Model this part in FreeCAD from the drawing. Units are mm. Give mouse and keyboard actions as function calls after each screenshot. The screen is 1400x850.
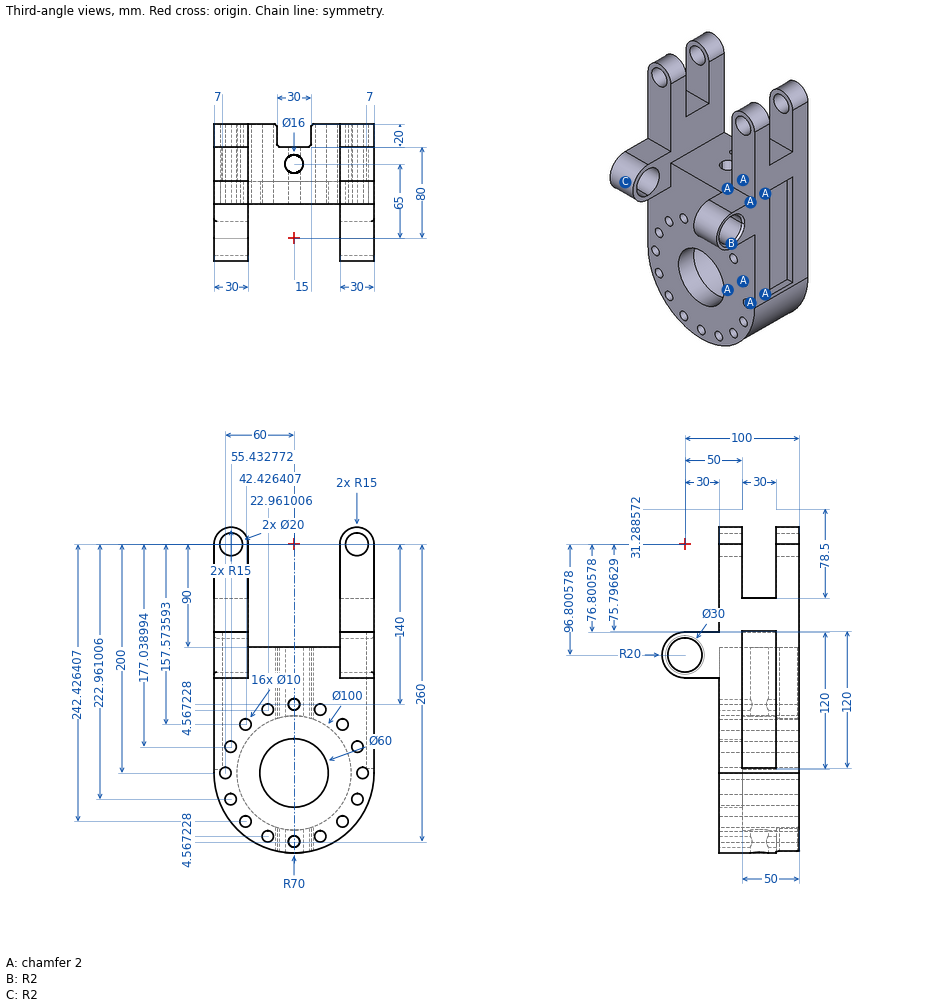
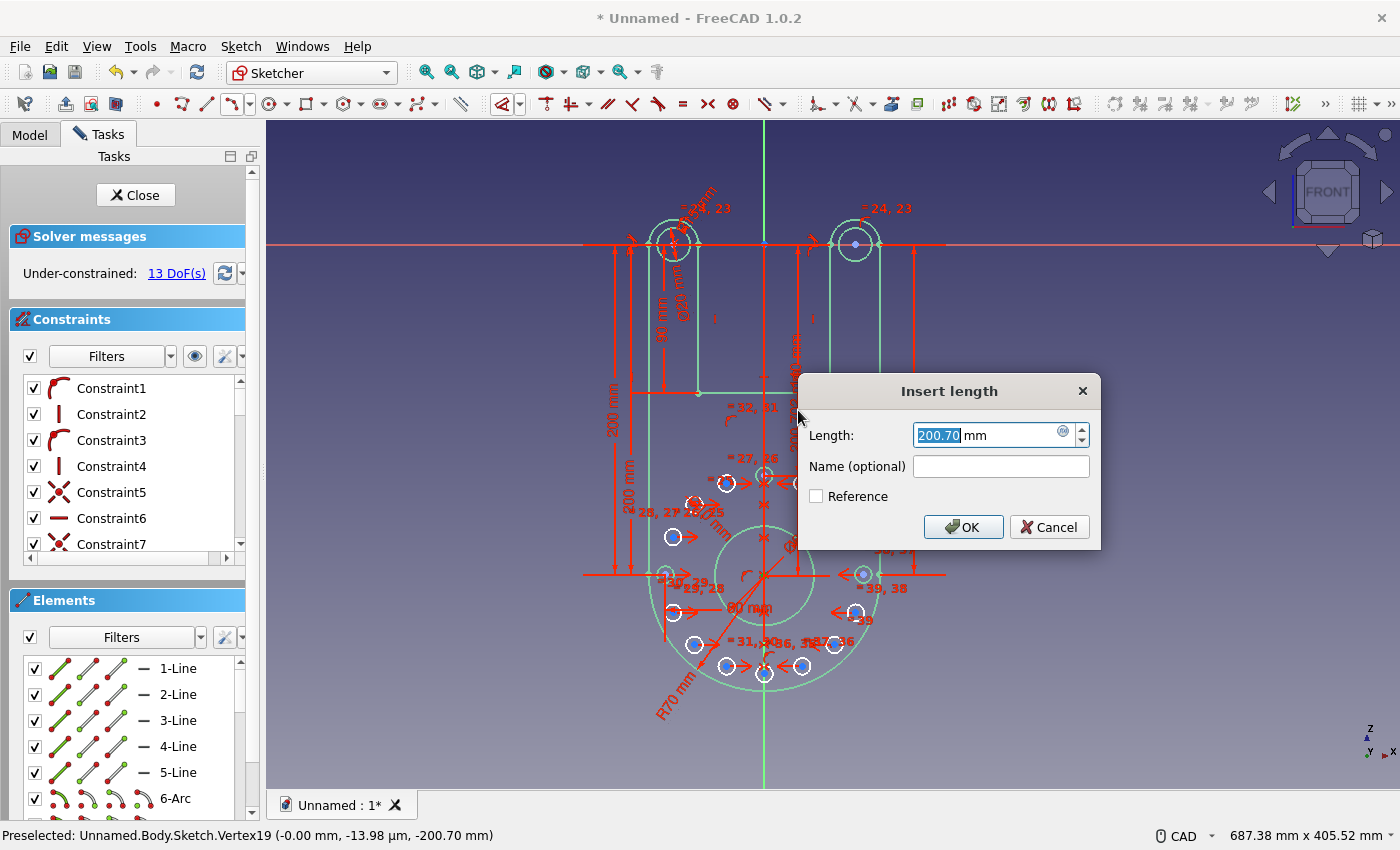
text(200)
key(Return)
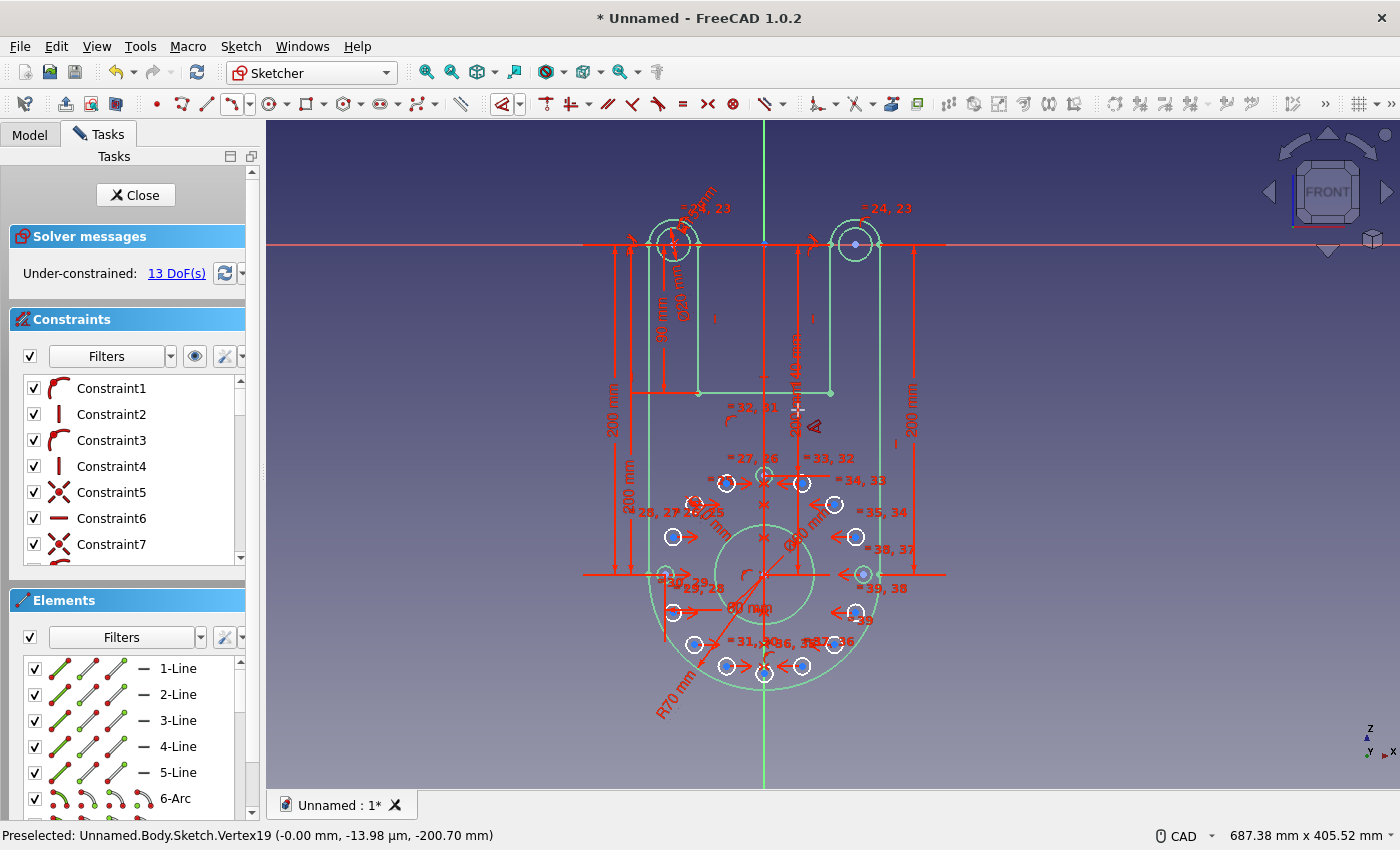
click(764, 674)
click(798, 459)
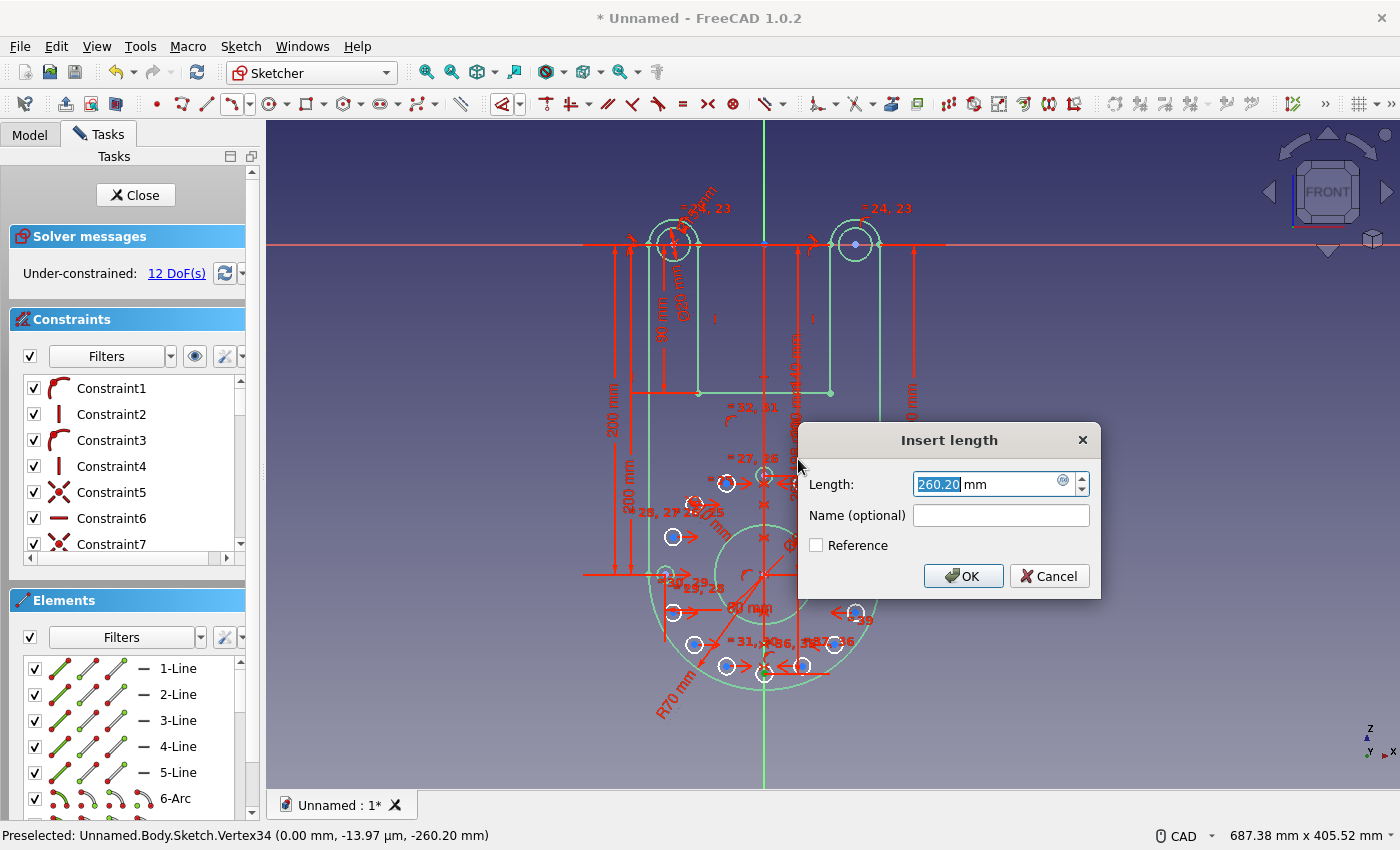
text(260)
key(Return)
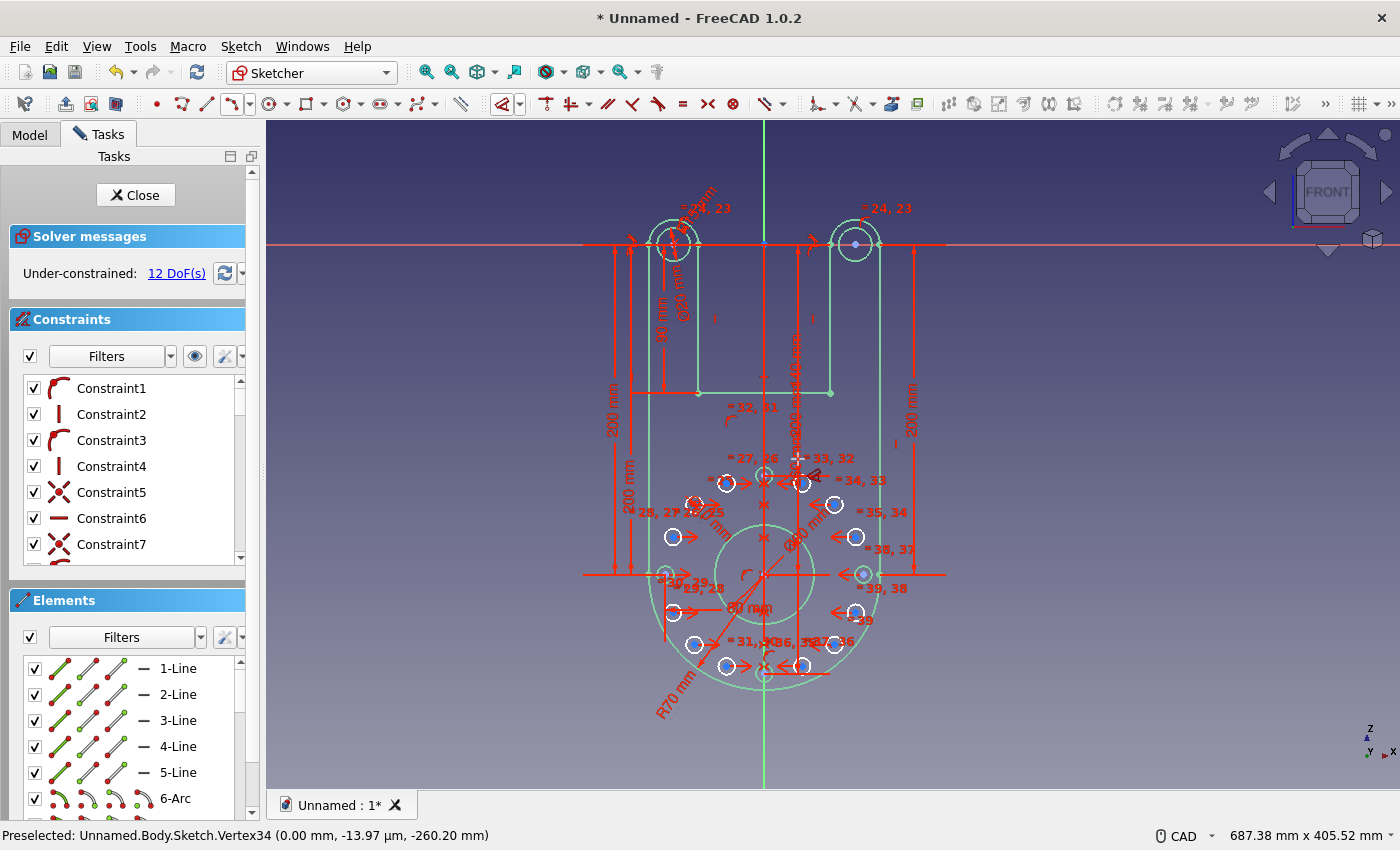
click(694, 505)
click(729, 187)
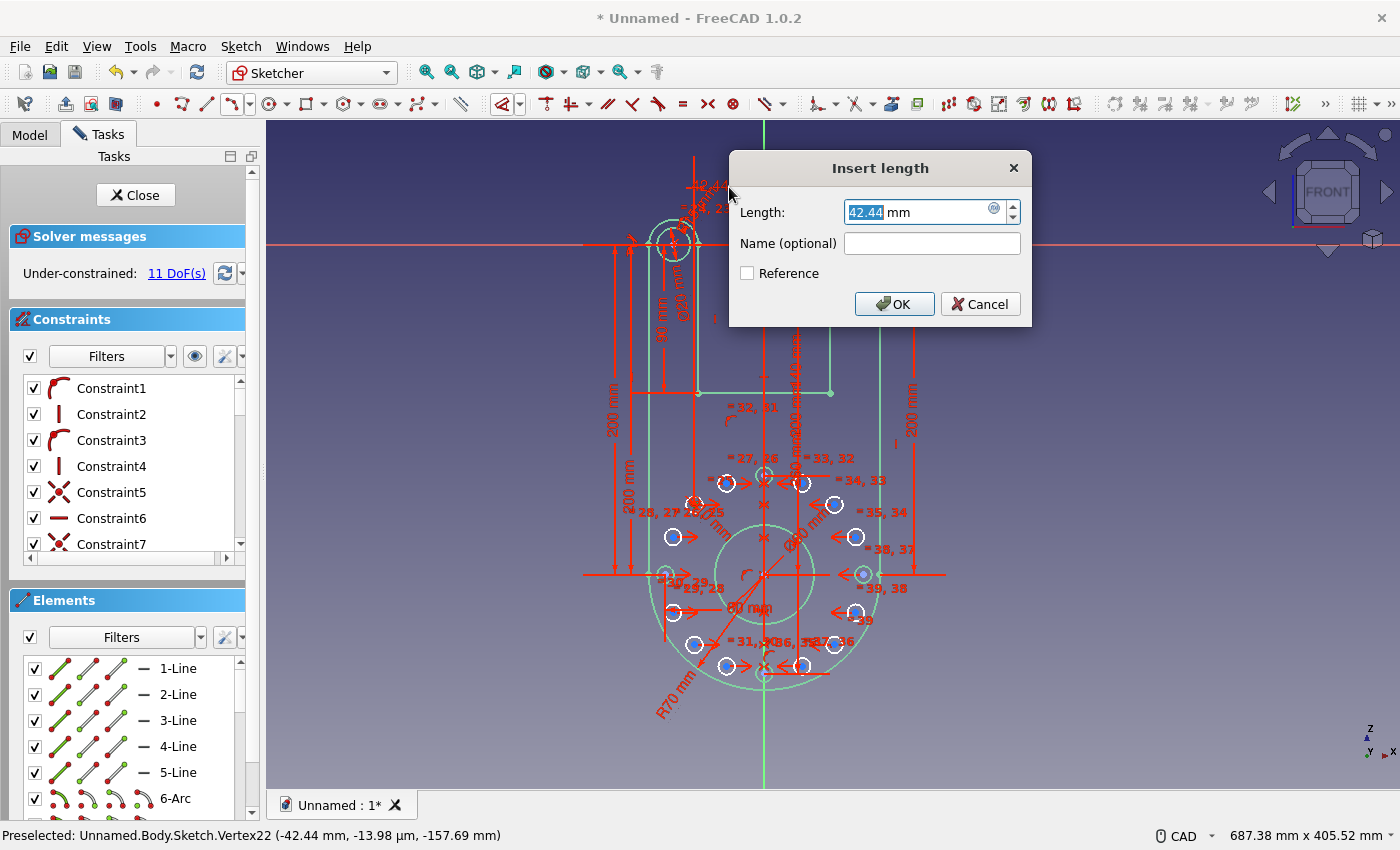
text(42.426407)
key(Return)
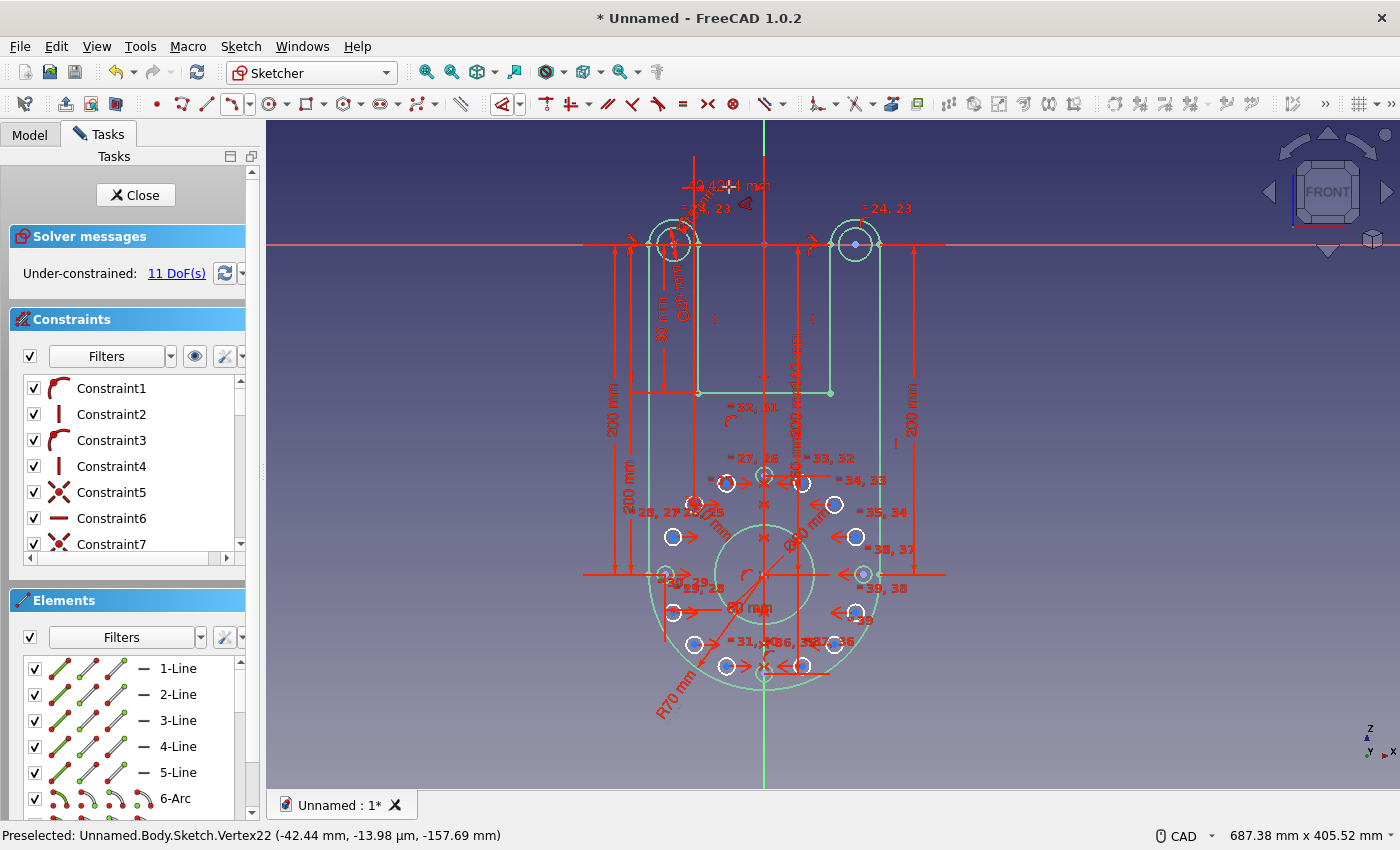
click(673, 537)
click(698, 571)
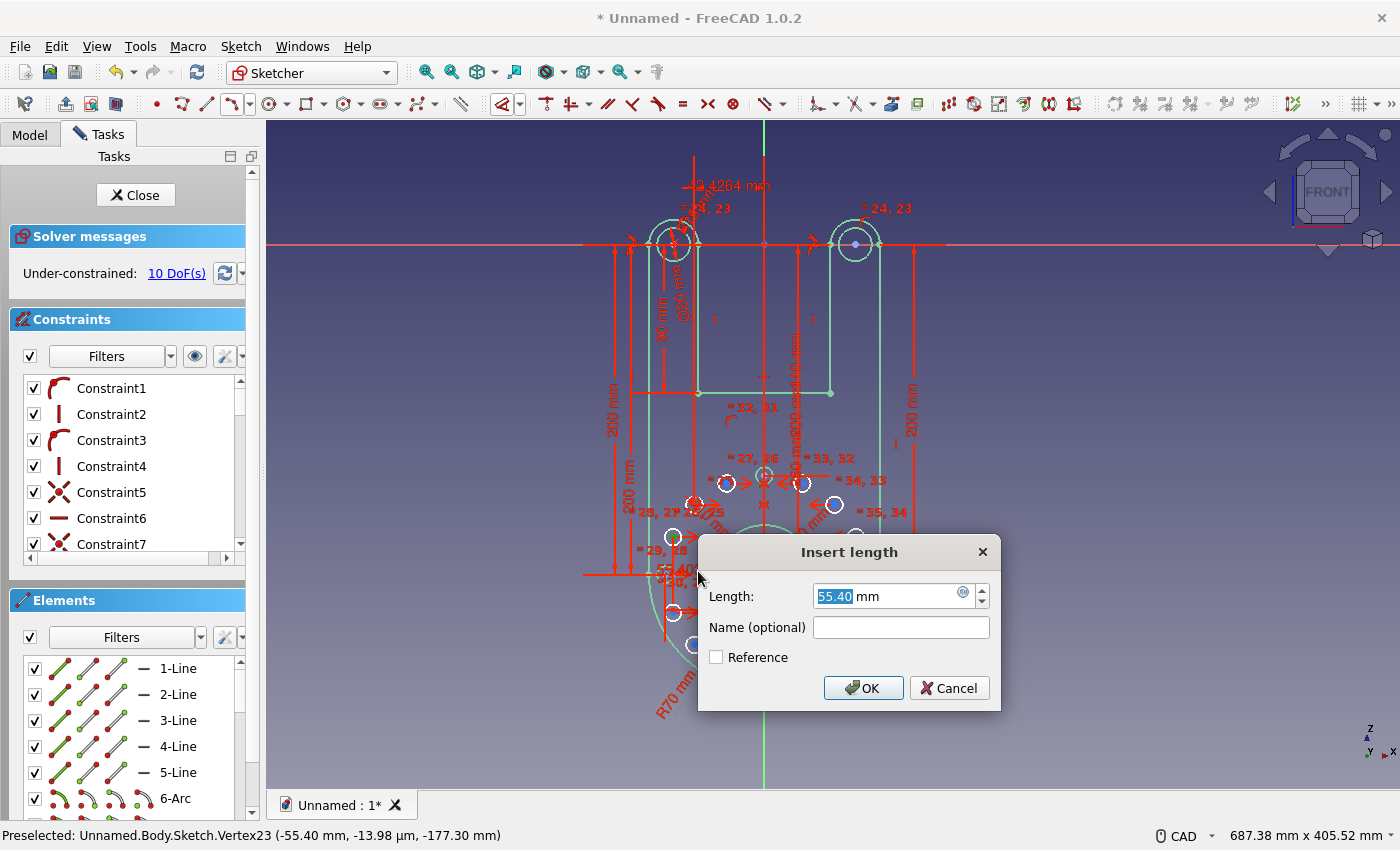
text(55.432772)
key(Return)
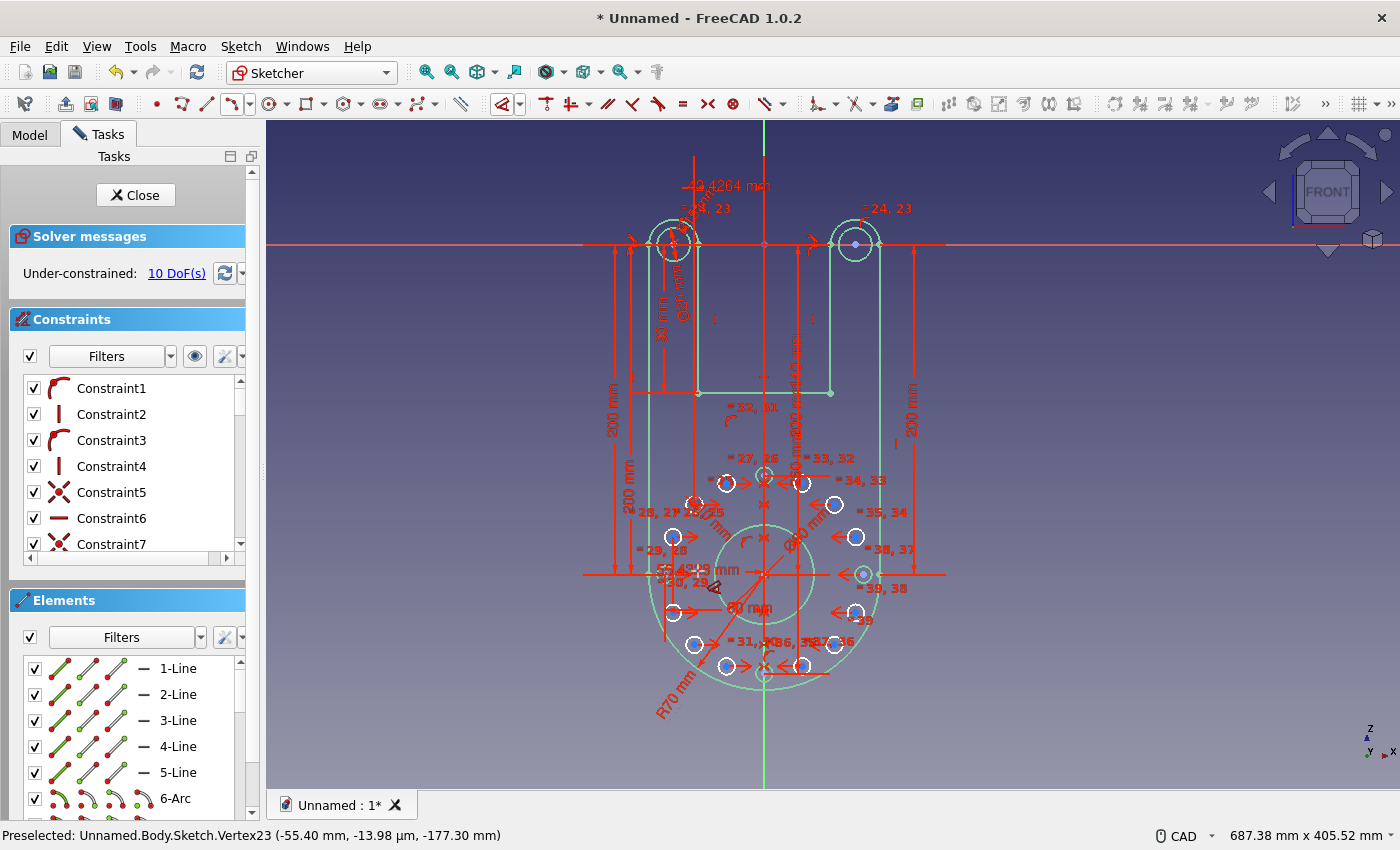
click(727, 484)
click(746, 163)